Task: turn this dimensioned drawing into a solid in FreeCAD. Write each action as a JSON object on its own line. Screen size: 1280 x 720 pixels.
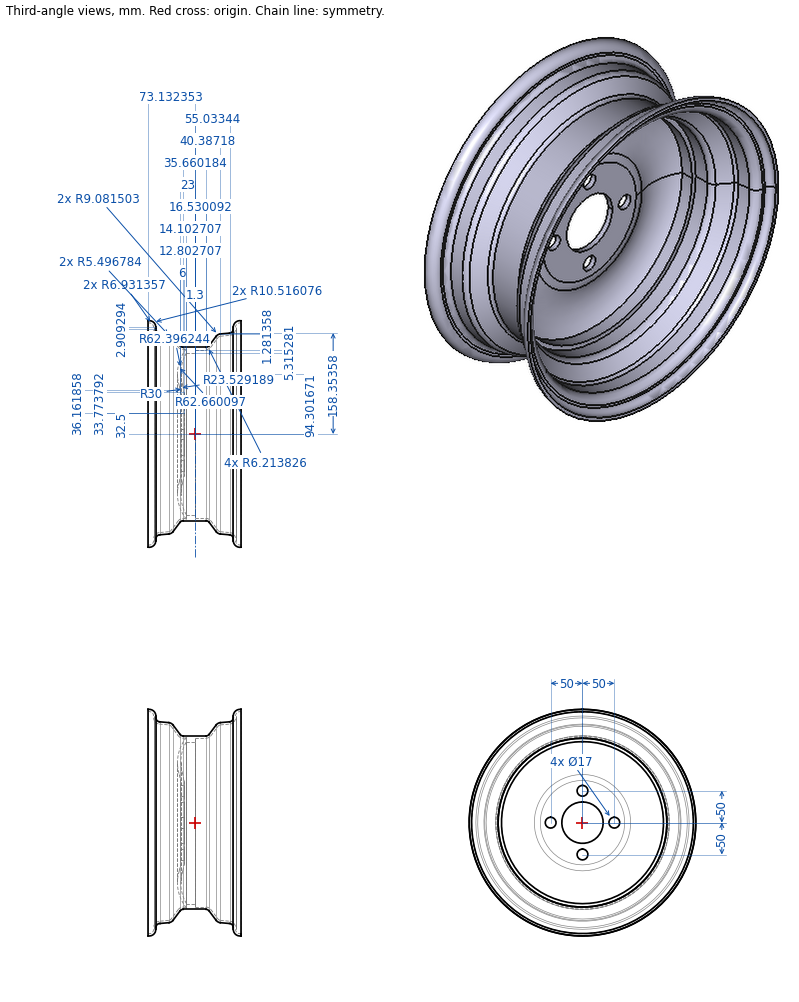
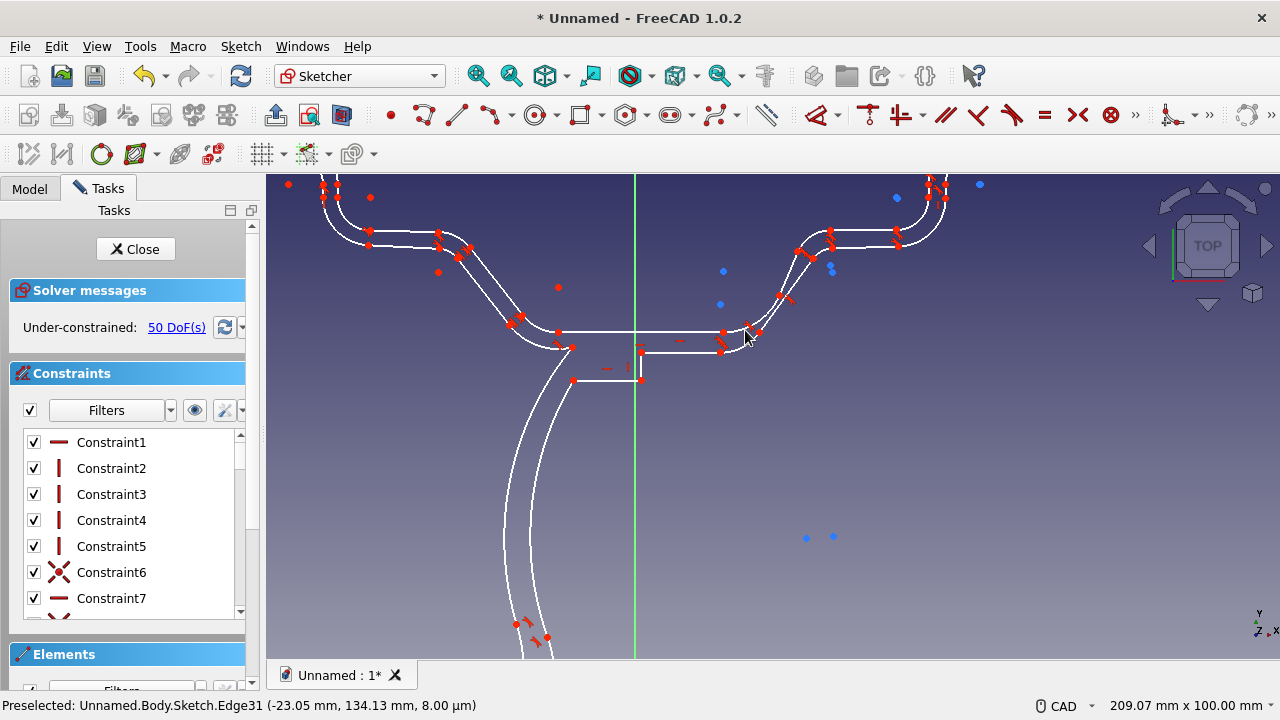
{"action": "left_click", "coordinate": [757, 322]}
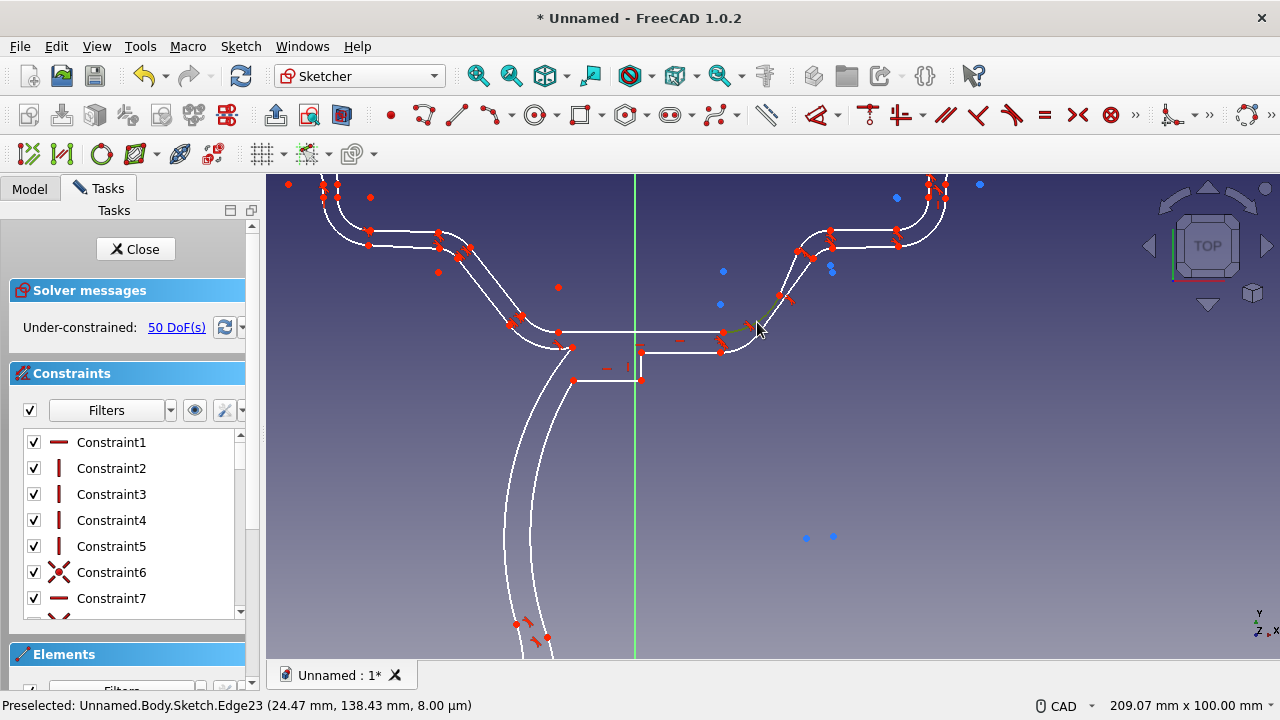
{"action": "left_click", "coordinate": [734, 351]}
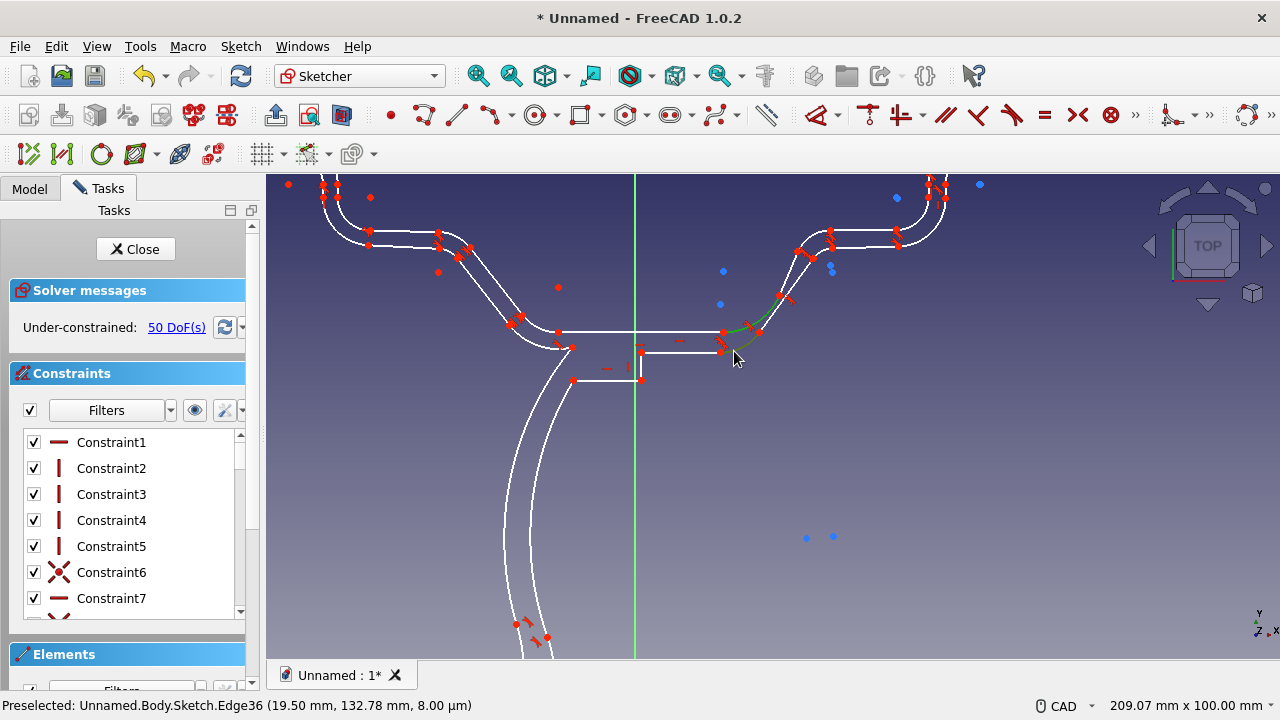
{"action": "key", "text": "c"}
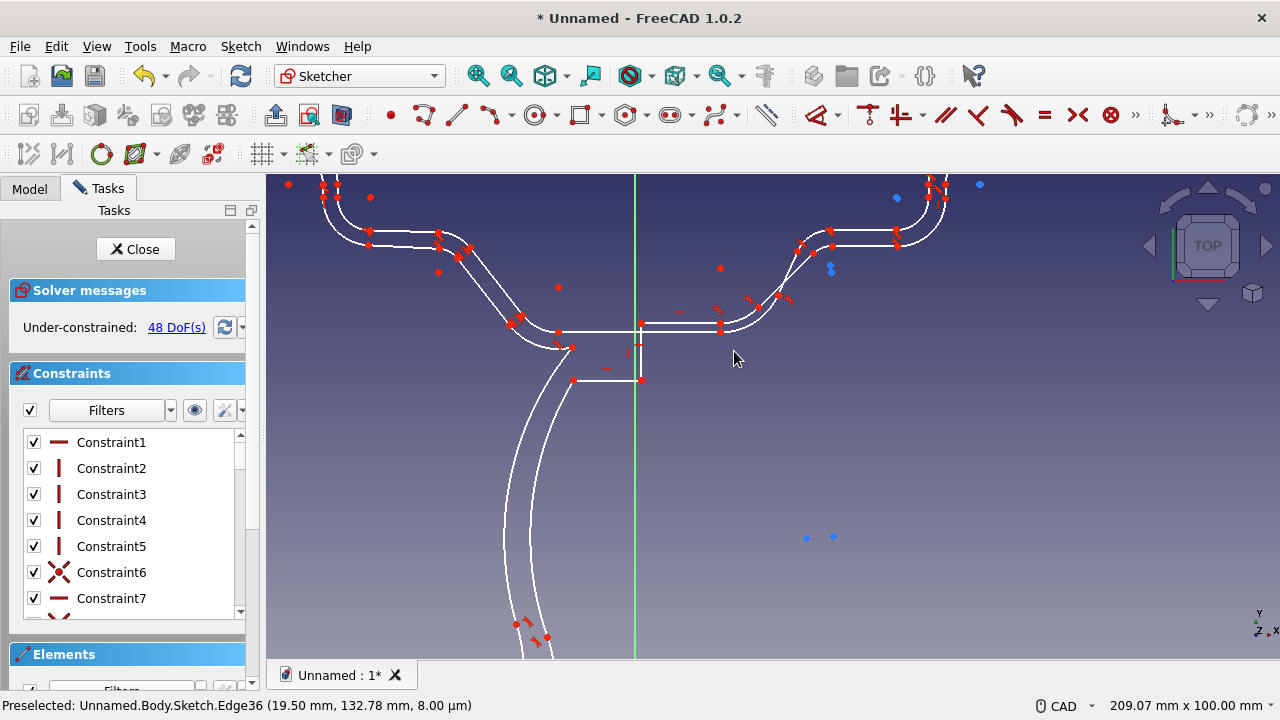
{"action": "left_click", "coordinate": [818, 232]}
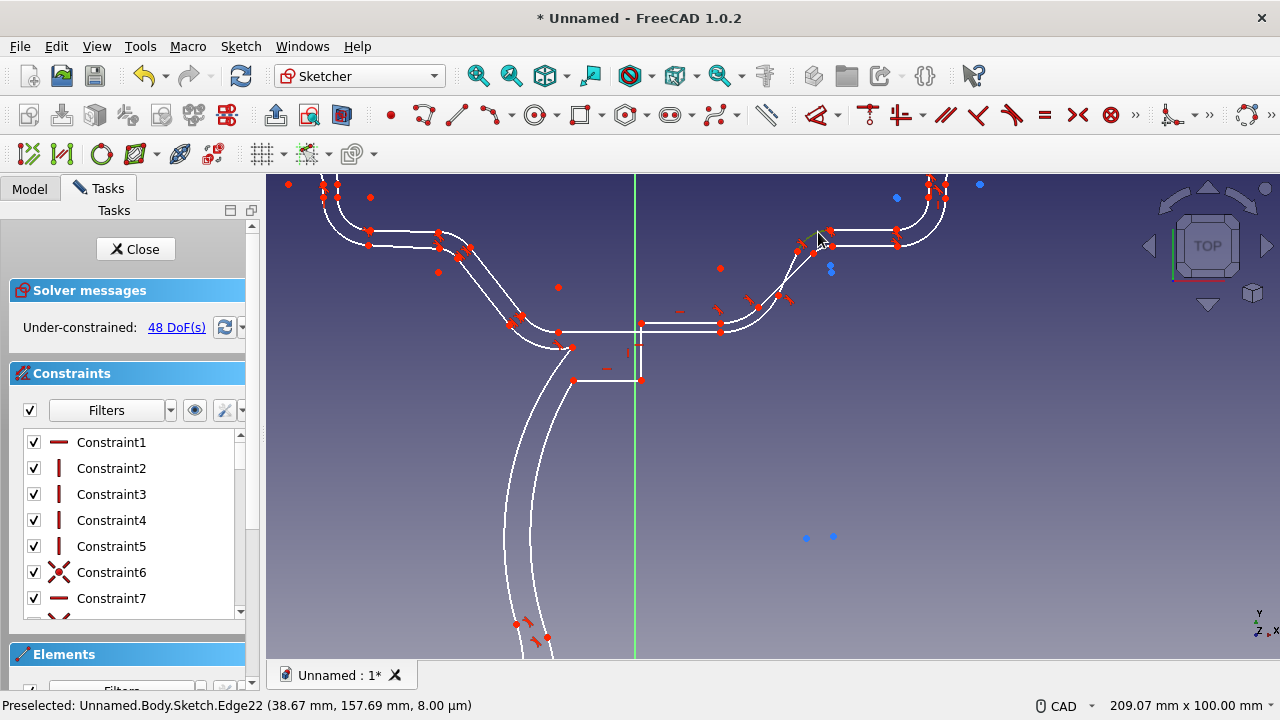
{"action": "scroll", "coordinate": [822, 248], "scroll_direction": "up", "scroll_amount": 2}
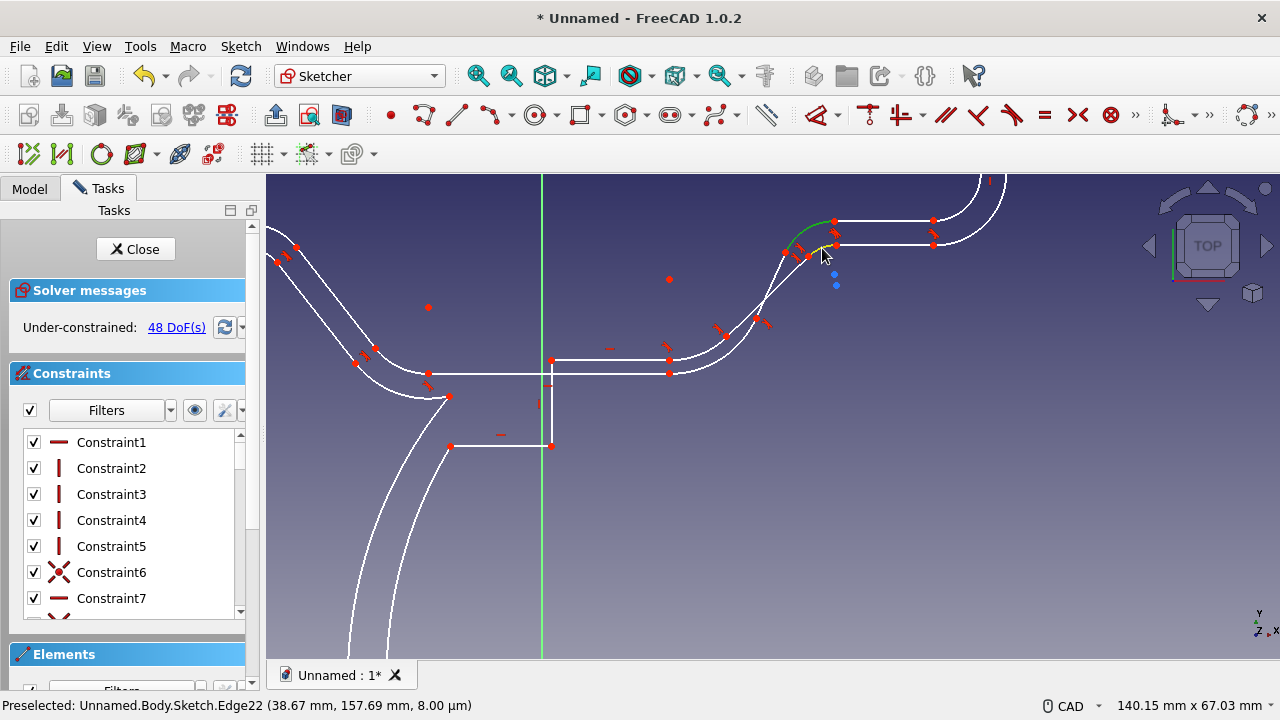
{"action": "left_click", "coordinate": [822, 248]}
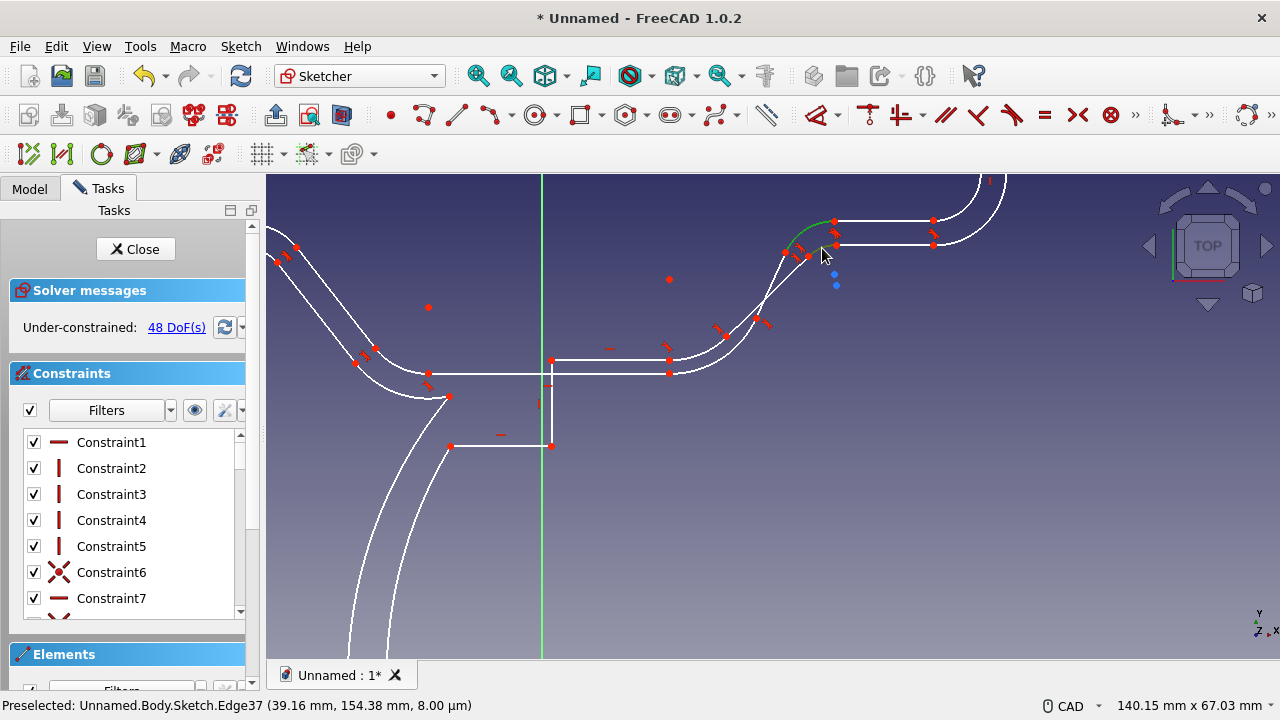
{"action": "left_click", "coordinate": [868, 116]}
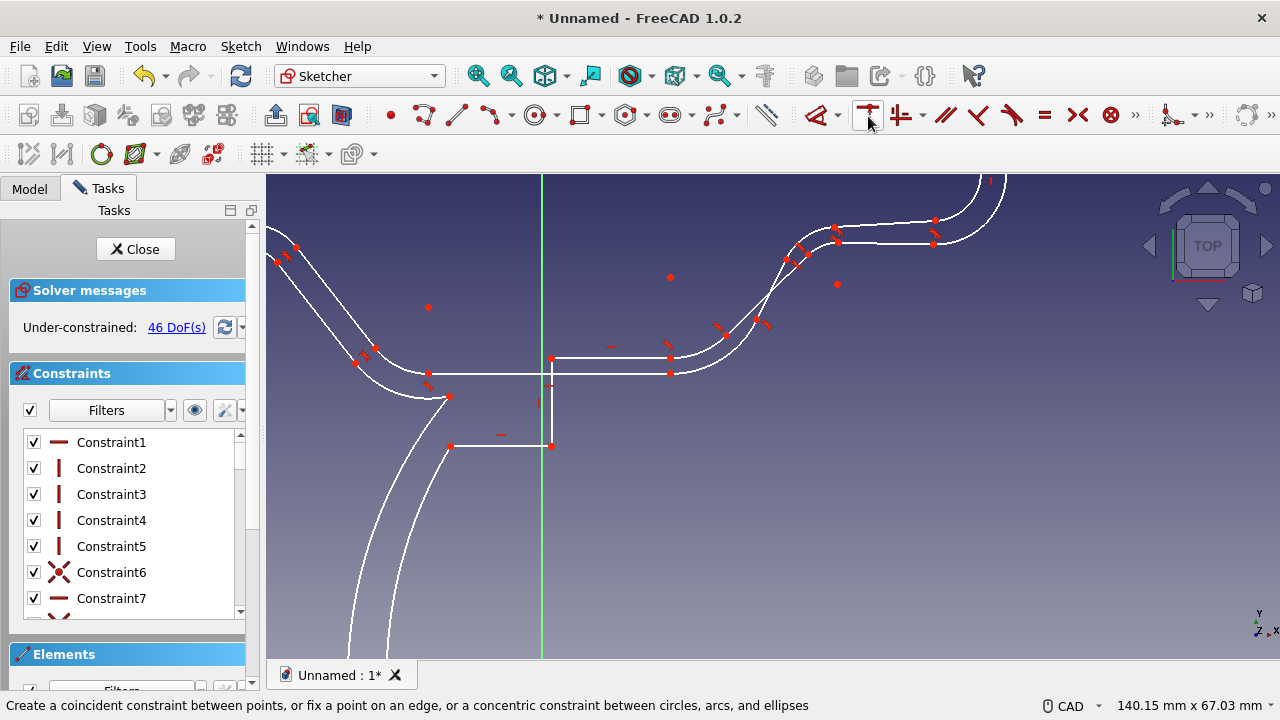
{"action": "scroll", "coordinate": [758, 317], "scroll_direction": "down", "scroll_amount": 7}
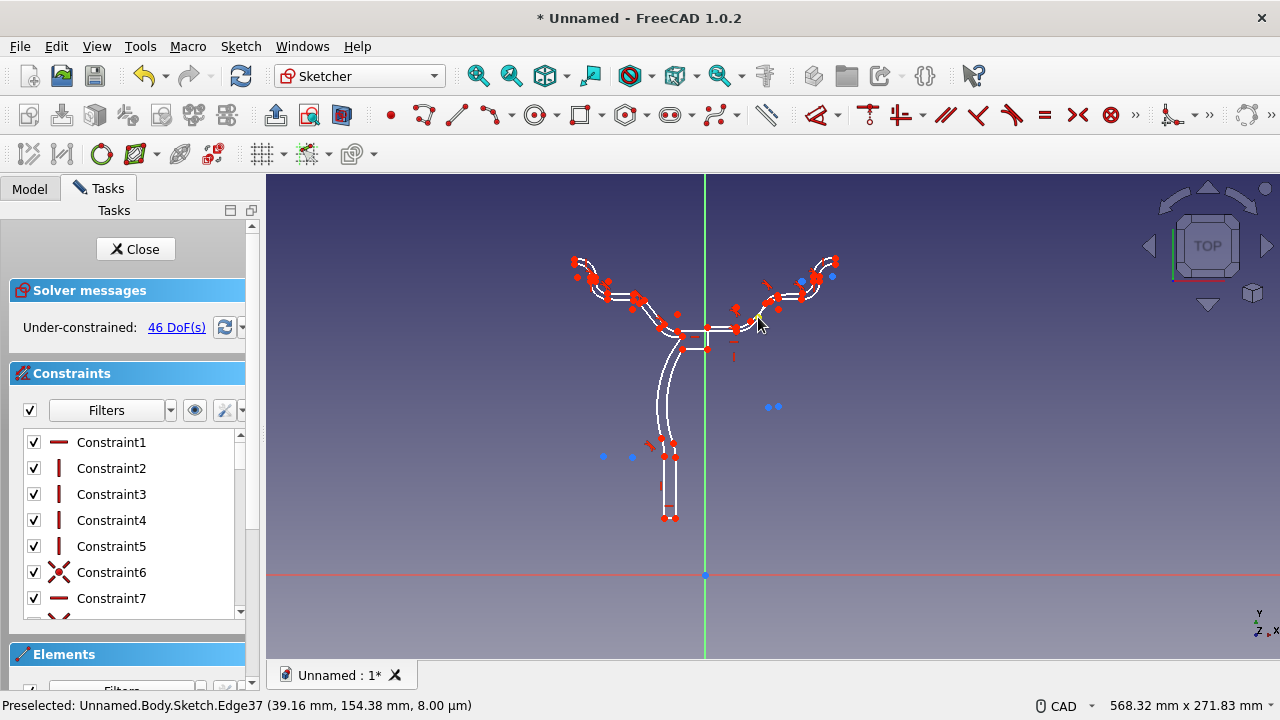
{"action": "scroll", "coordinate": [829, 265], "scroll_direction": "up", "scroll_amount": 4}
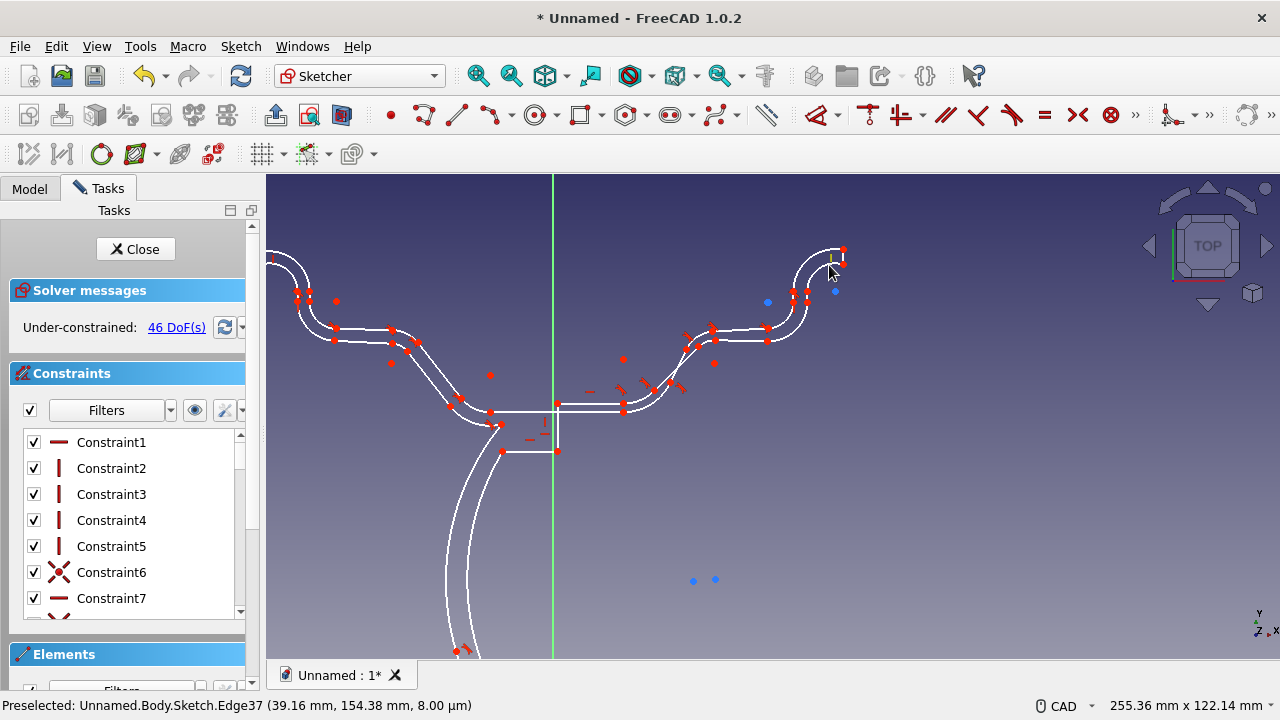
{"action": "left_click", "coordinate": [828, 264]}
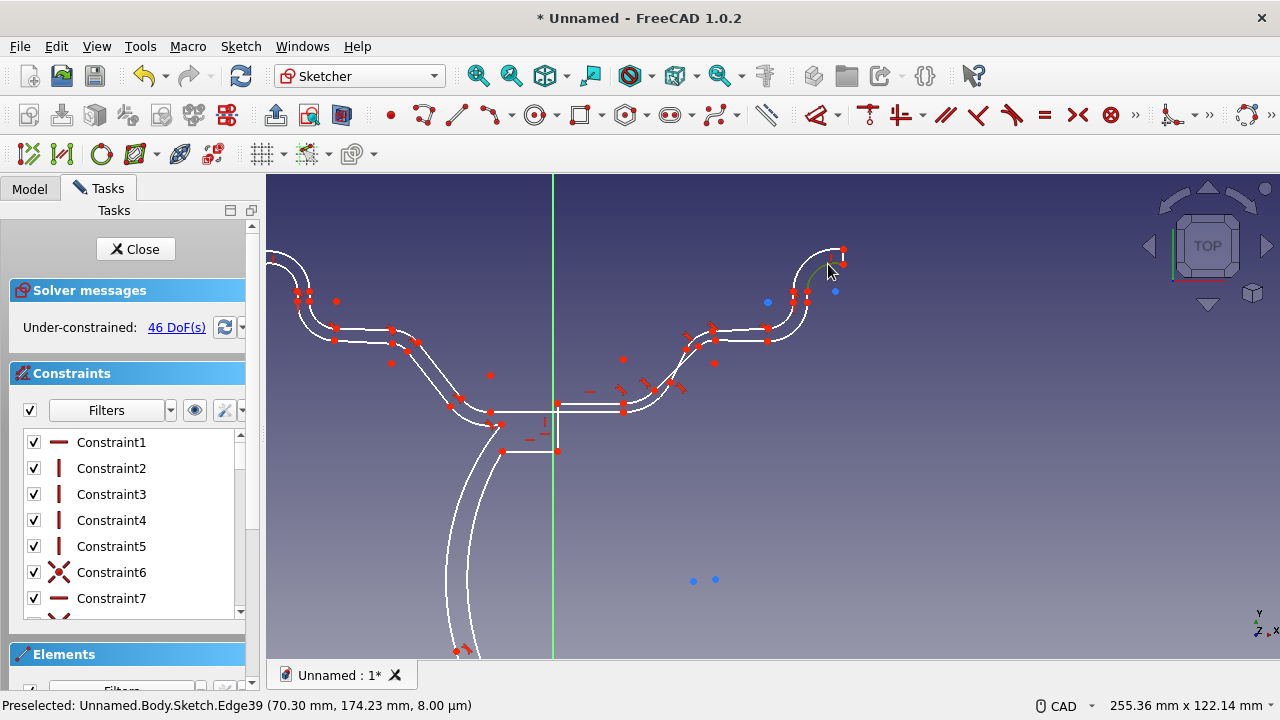
{"action": "left_click", "coordinate": [821, 252]}